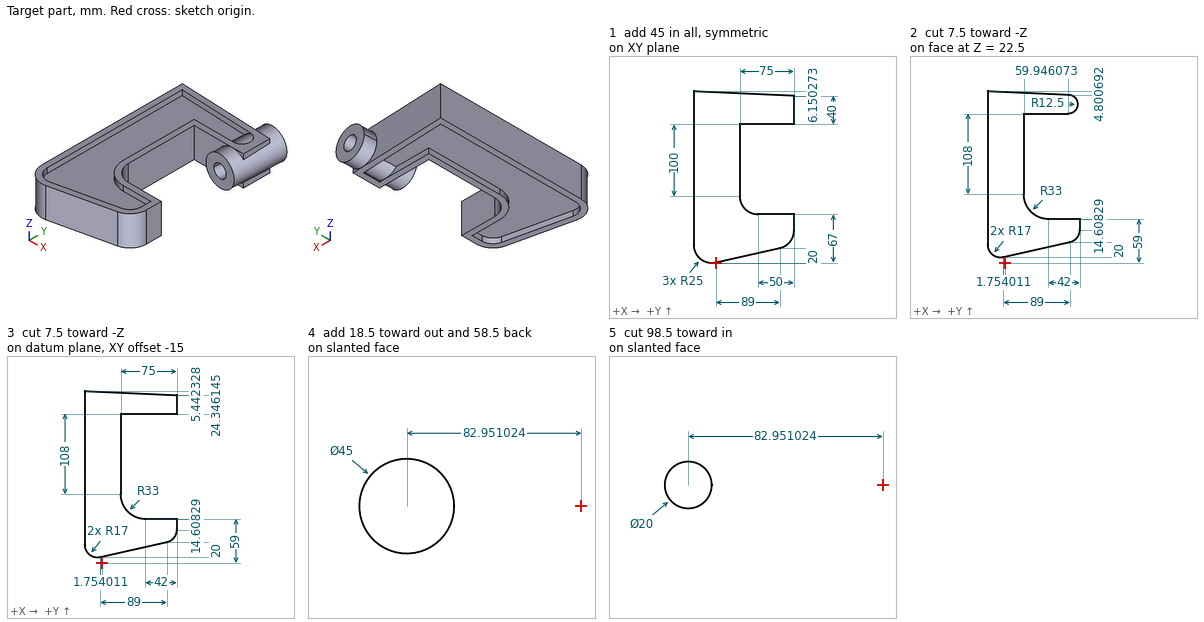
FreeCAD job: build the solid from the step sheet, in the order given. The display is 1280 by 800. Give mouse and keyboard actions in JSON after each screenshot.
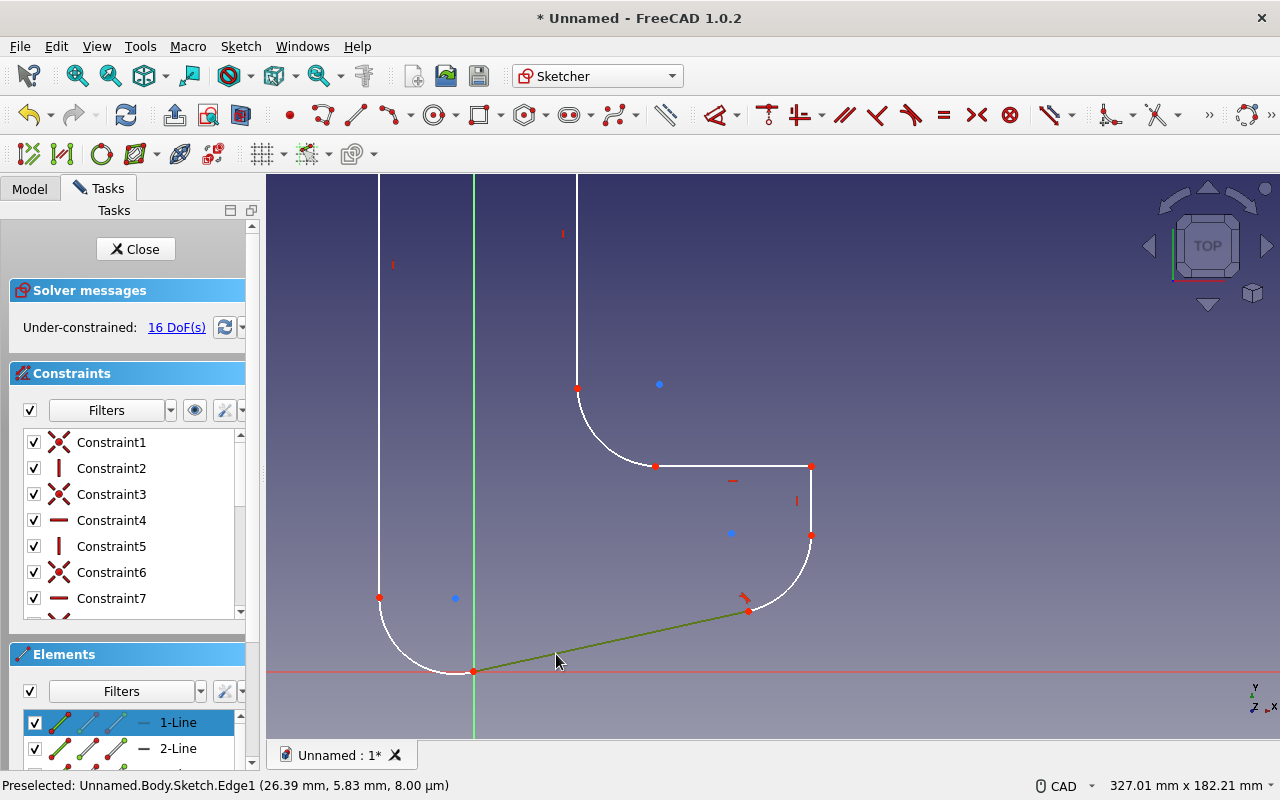
{"action": "left_click", "coordinate": [390, 637]}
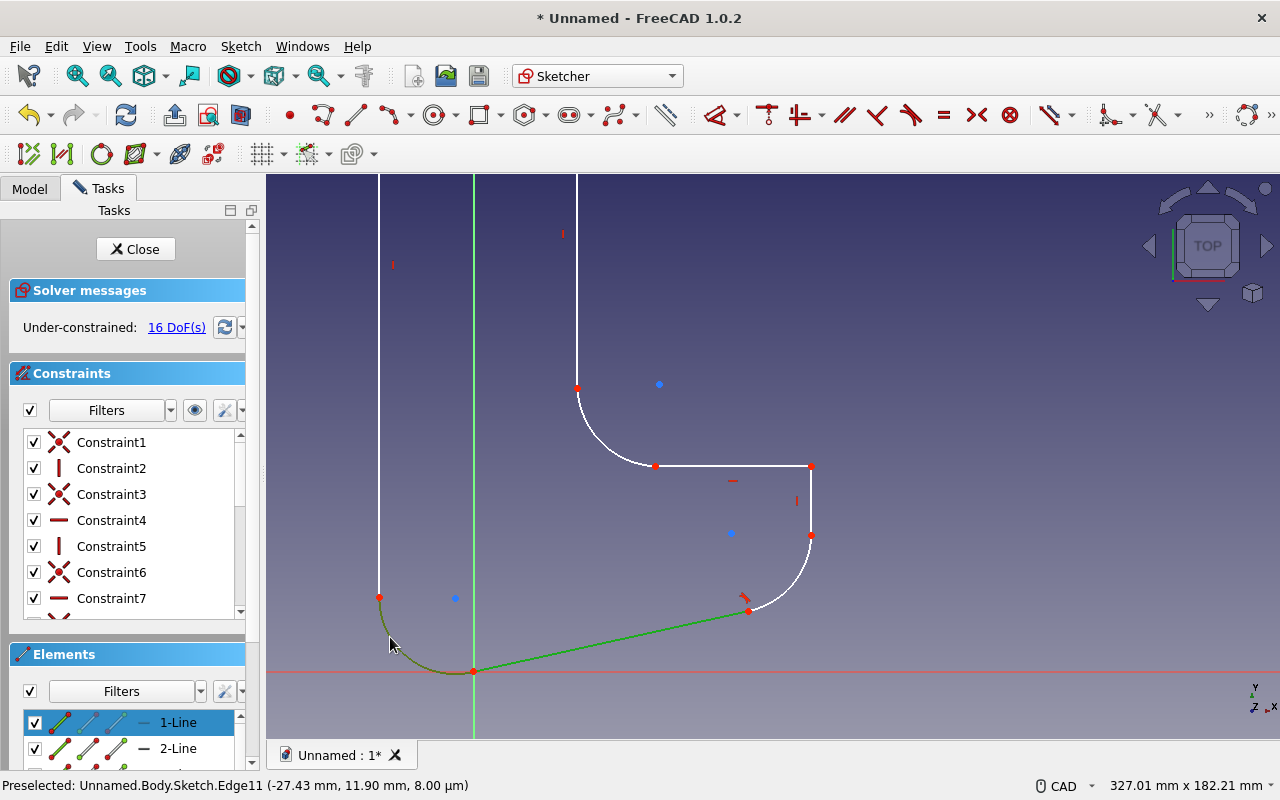
{"action": "left_click", "coordinate": [911, 116]}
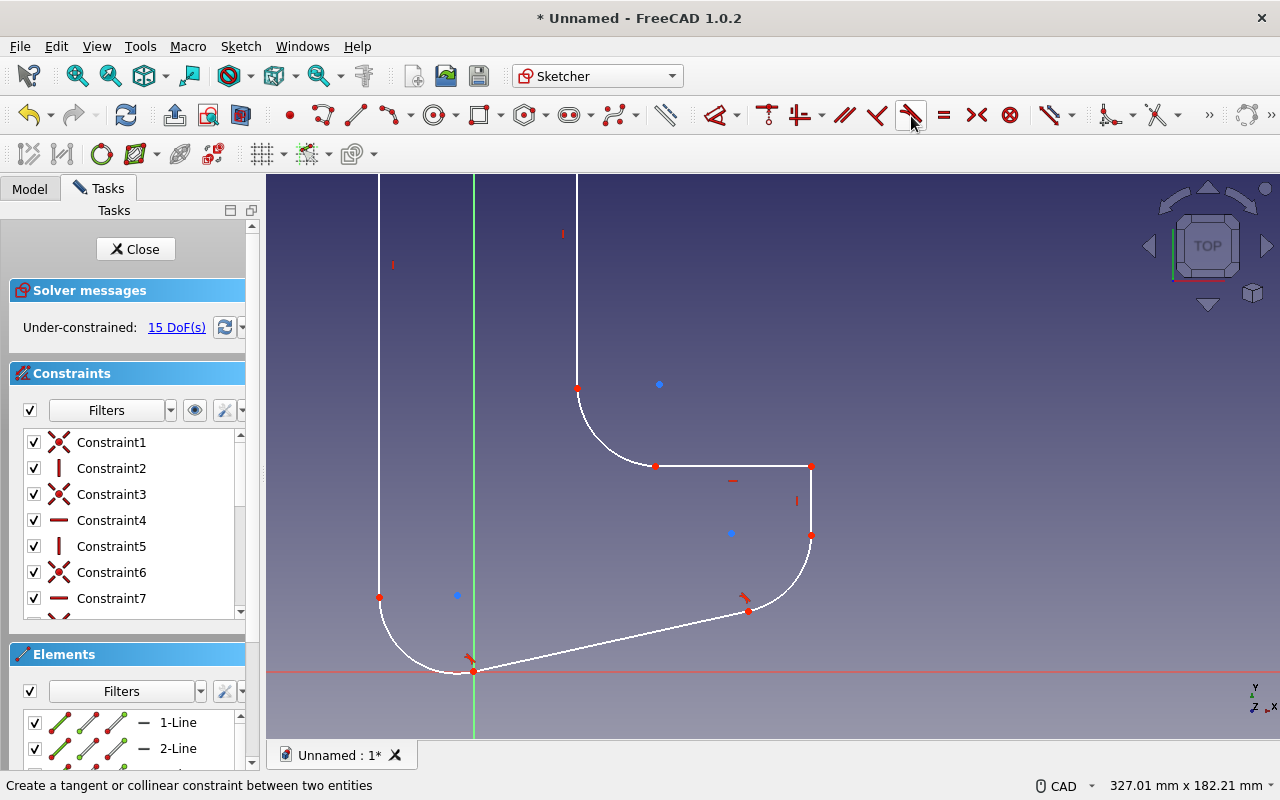
{"action": "left_click", "coordinate": [811, 515]}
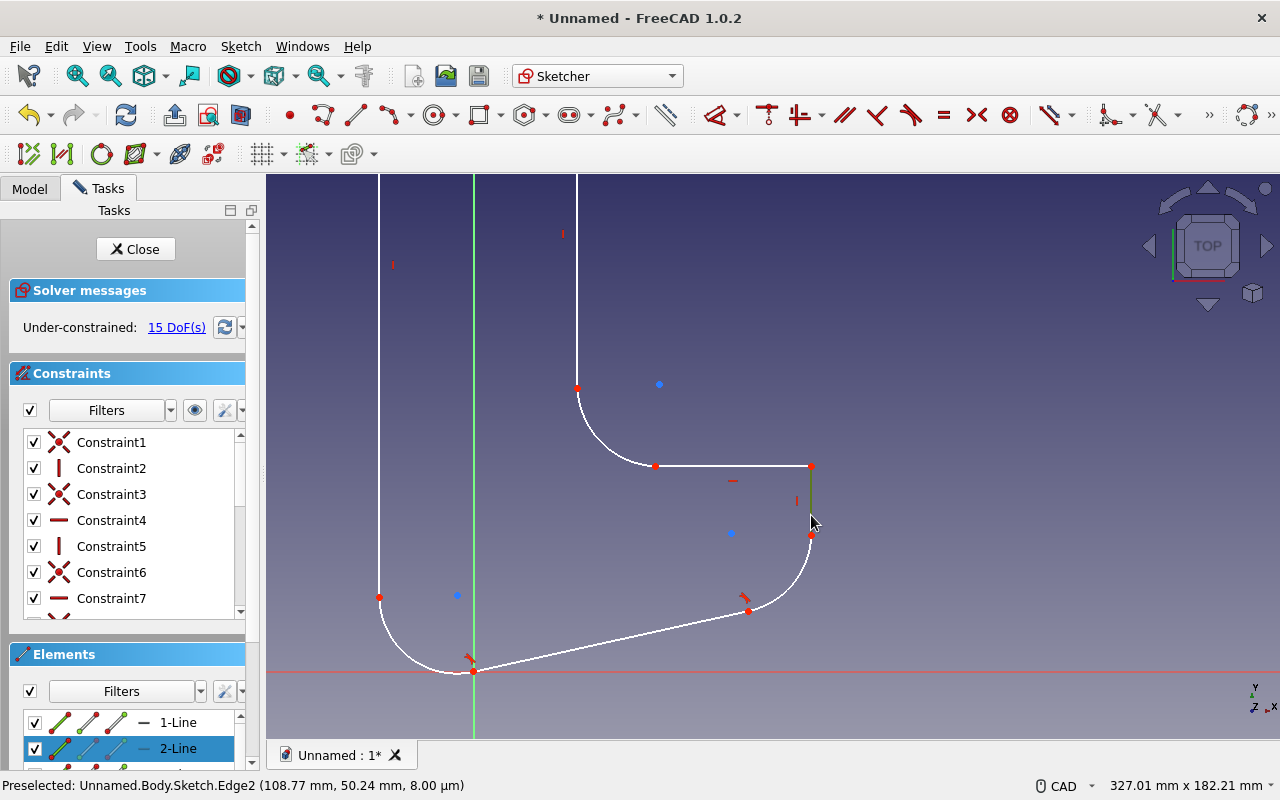
{"action": "left_click", "coordinate": [778, 598]}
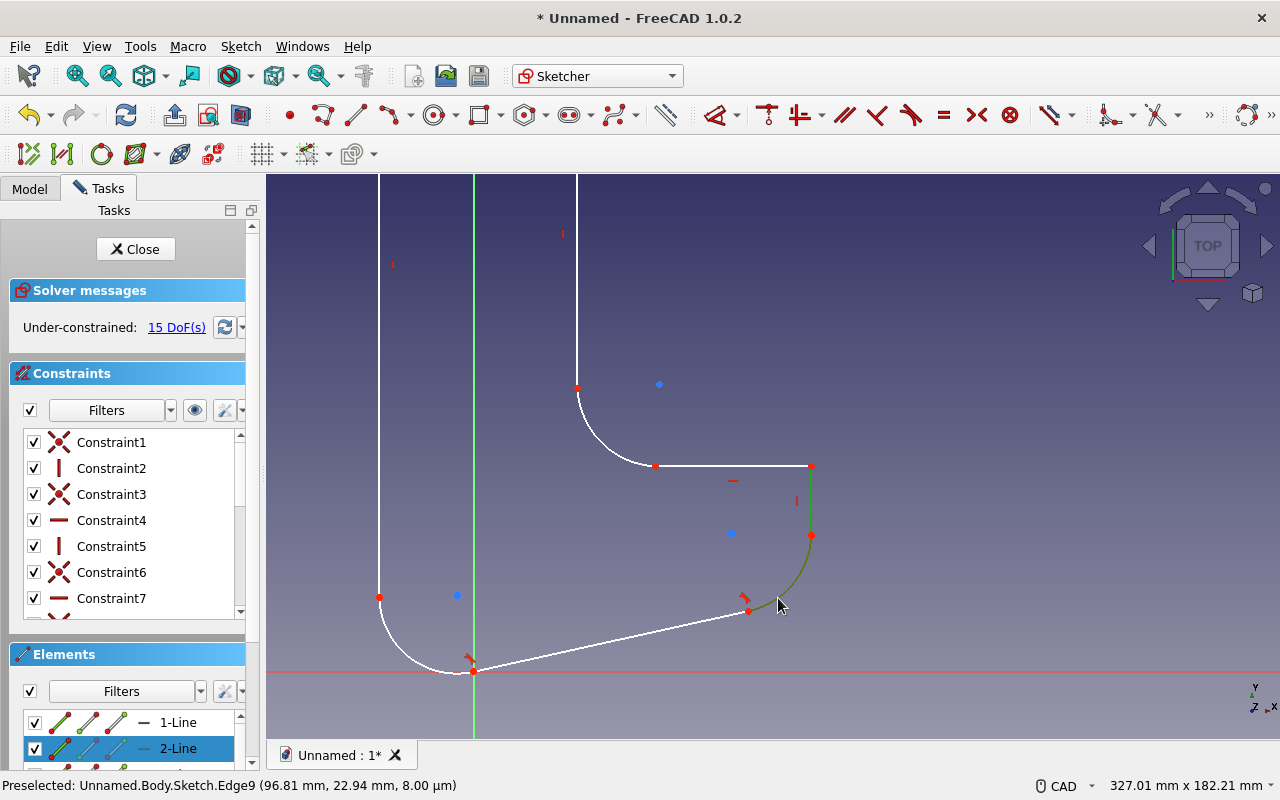
{"action": "left_click", "coordinate": [911, 116]}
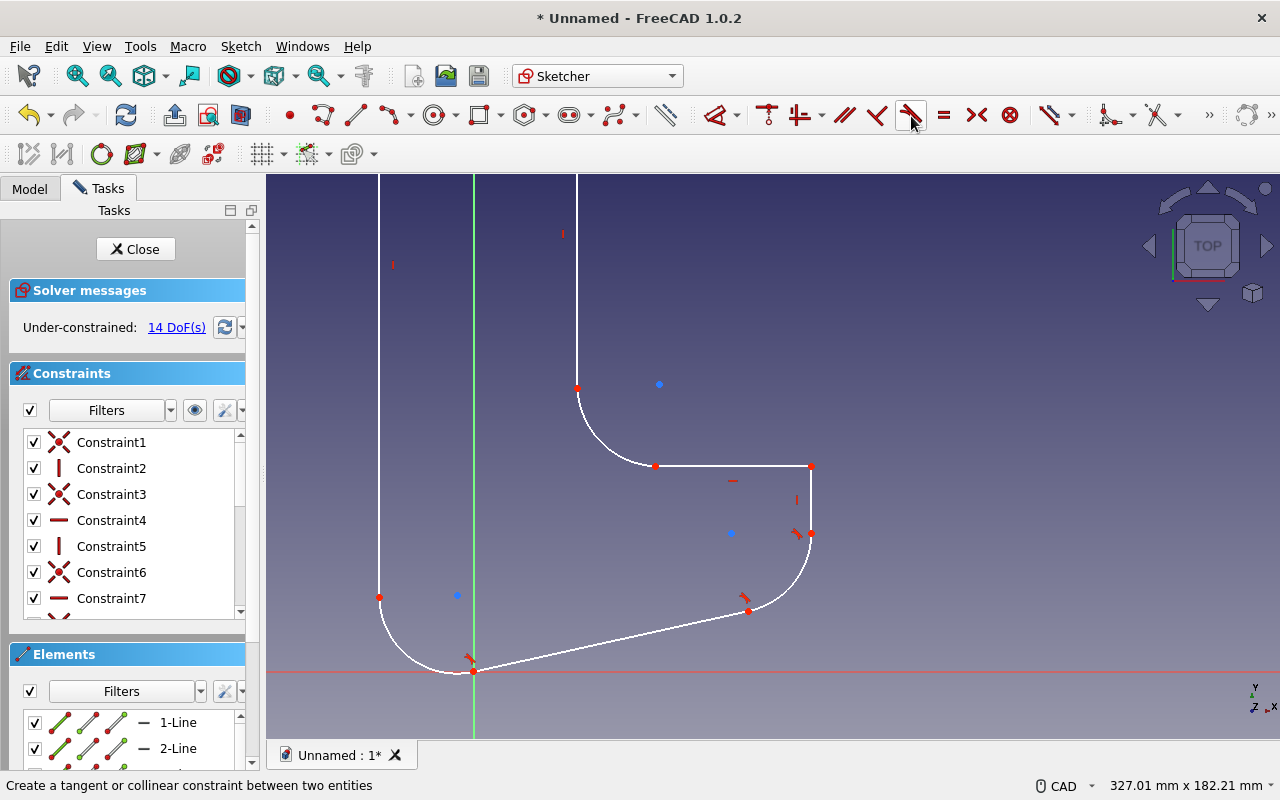
{"action": "left_click", "coordinate": [764, 466]}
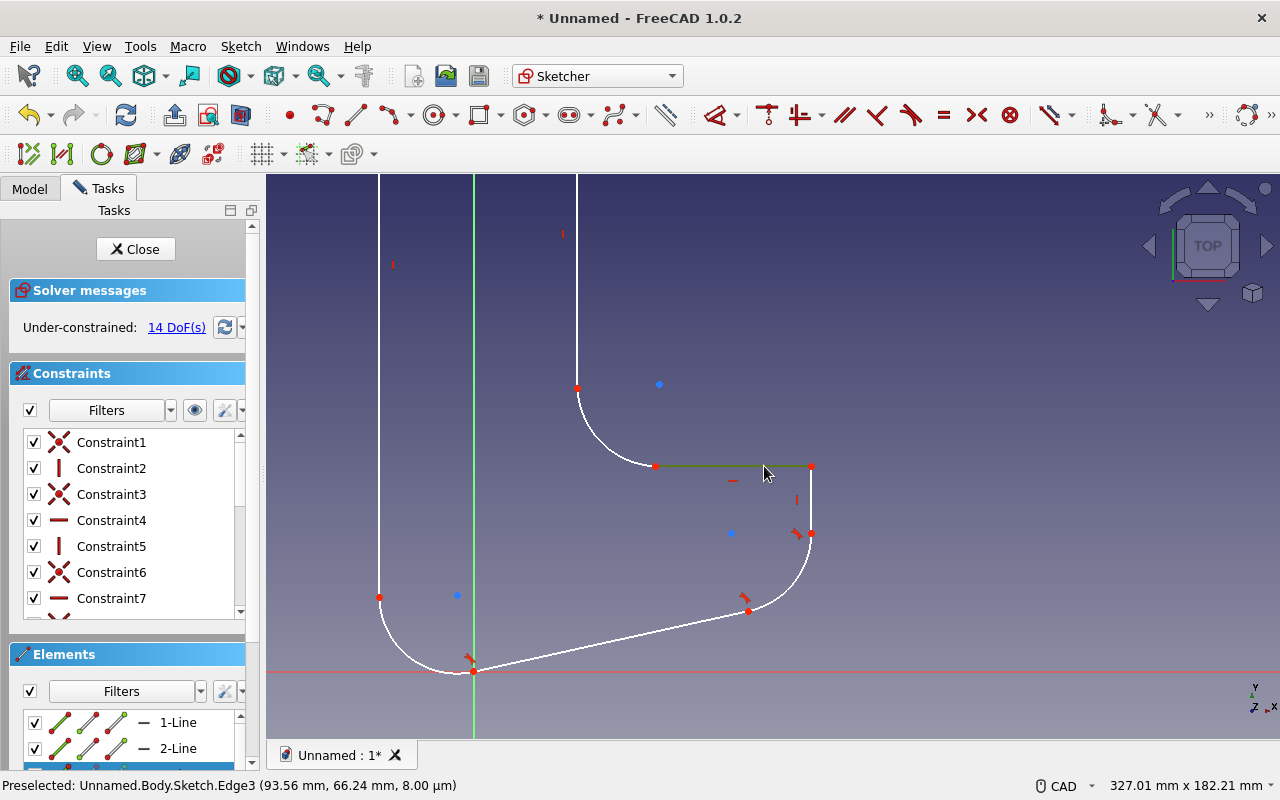
{"action": "left_click", "coordinate": [587, 423]}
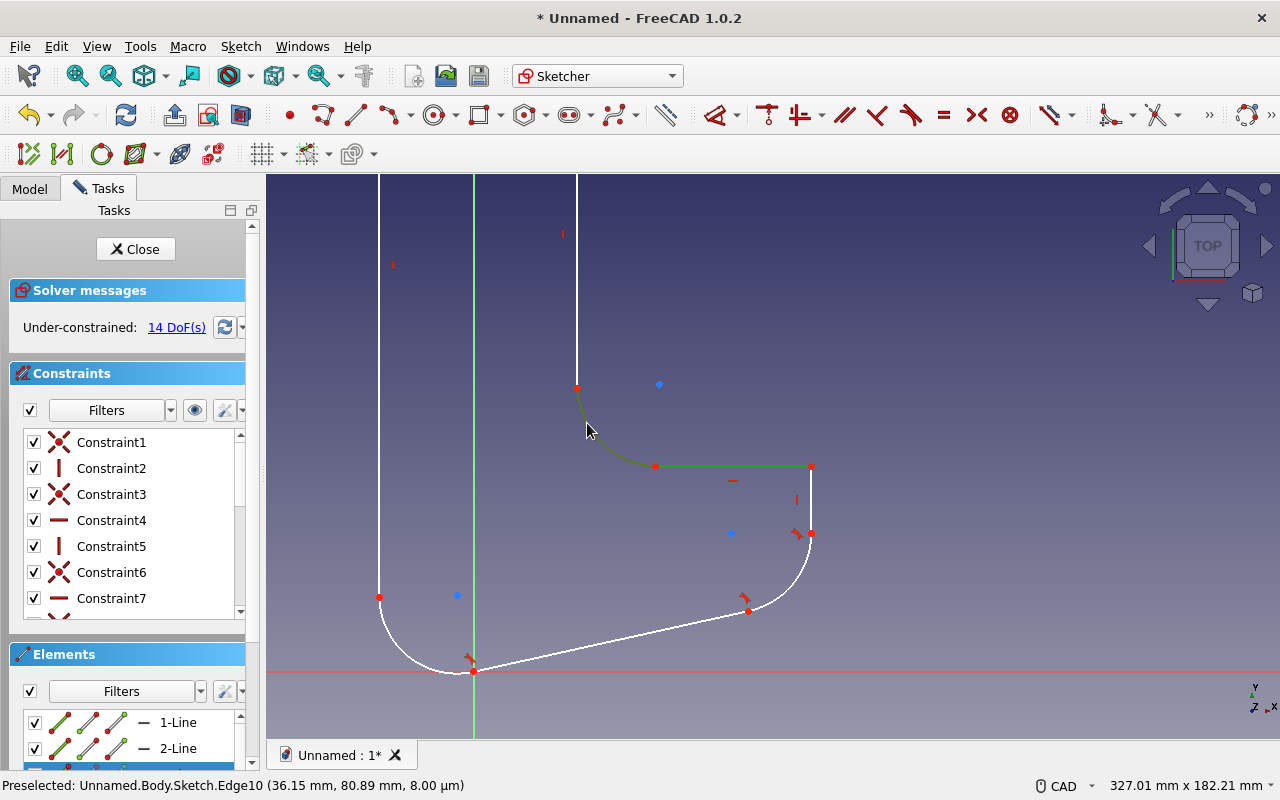
{"action": "left_click", "coordinate": [911, 116]}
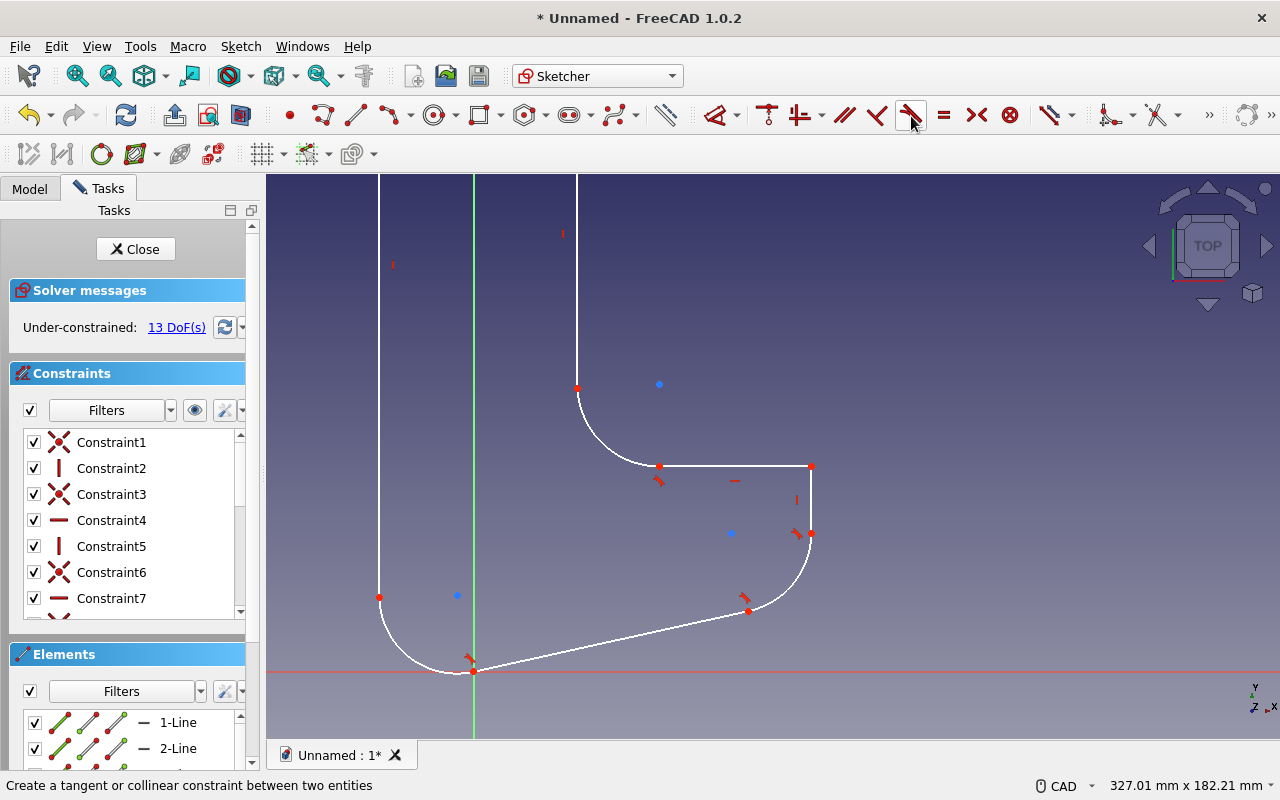
{"action": "left_click", "coordinate": [577, 296]}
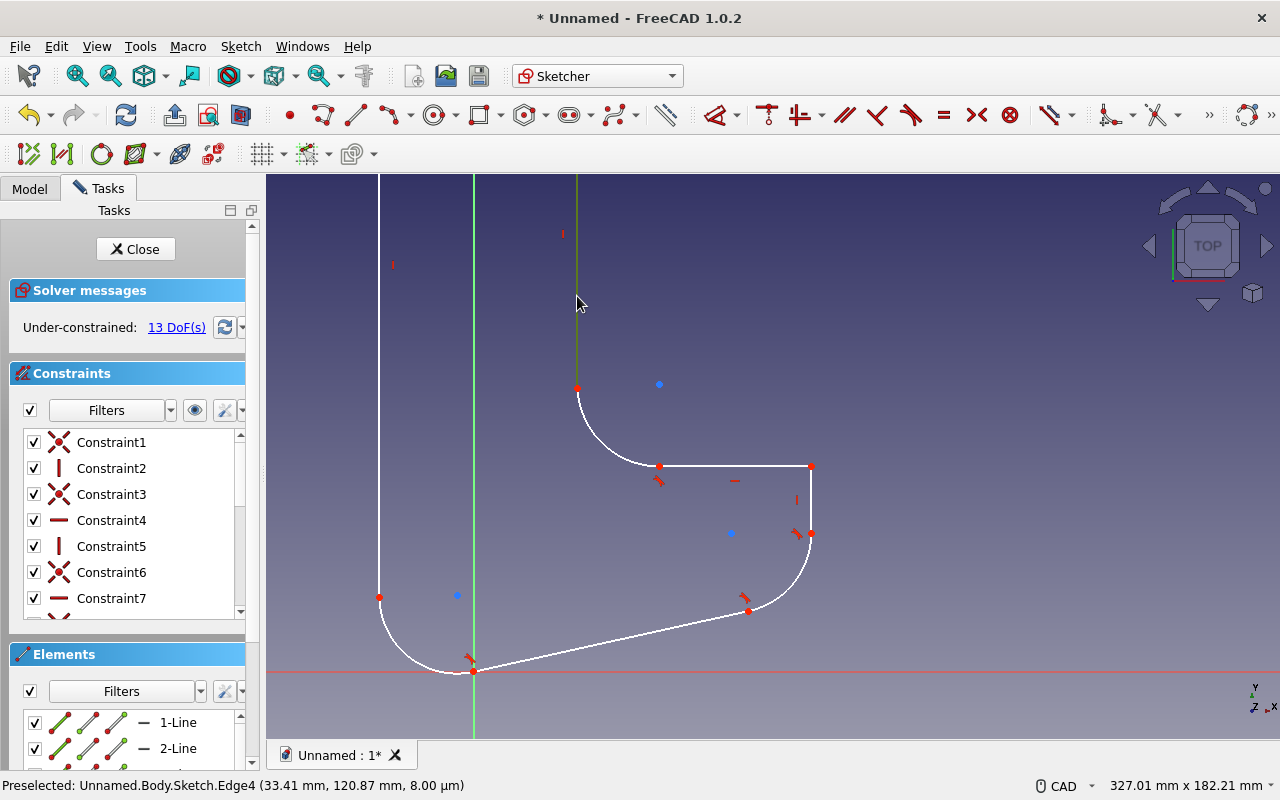
{"action": "left_click", "coordinate": [588, 424]}